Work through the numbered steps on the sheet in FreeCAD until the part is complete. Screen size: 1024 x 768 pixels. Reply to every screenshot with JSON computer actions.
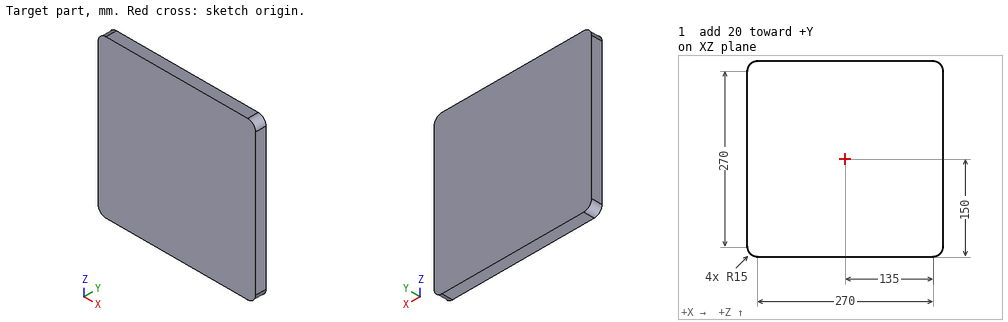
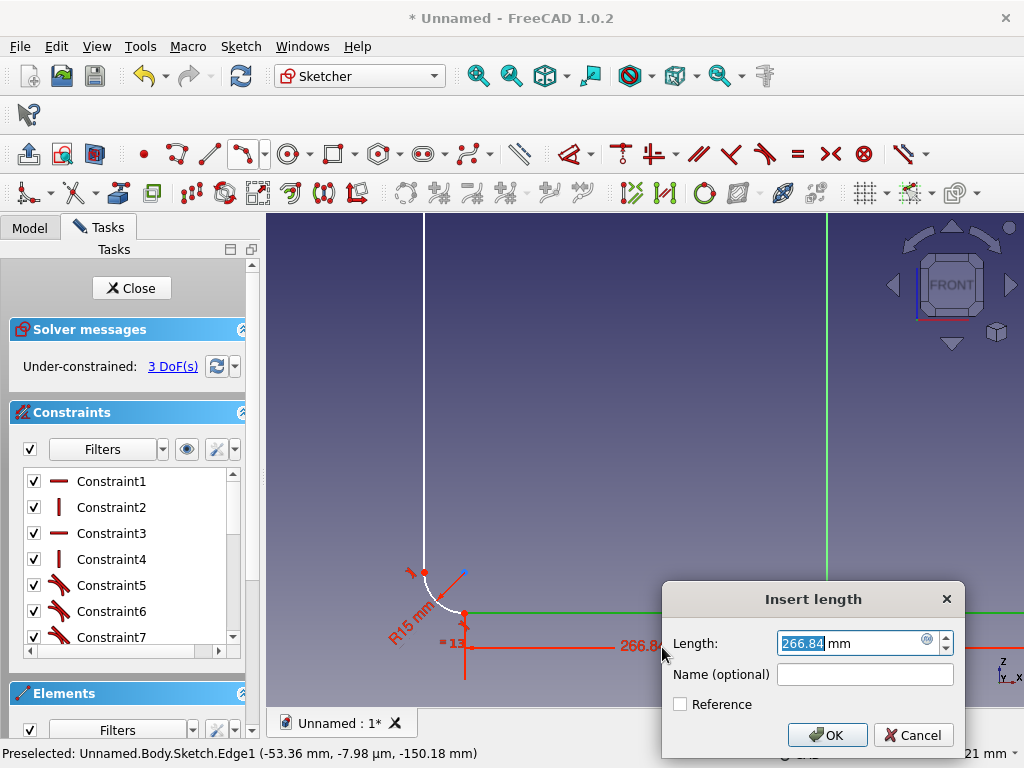
{"action": "type", "text": "270"}
{"action": "key", "text": "Return"}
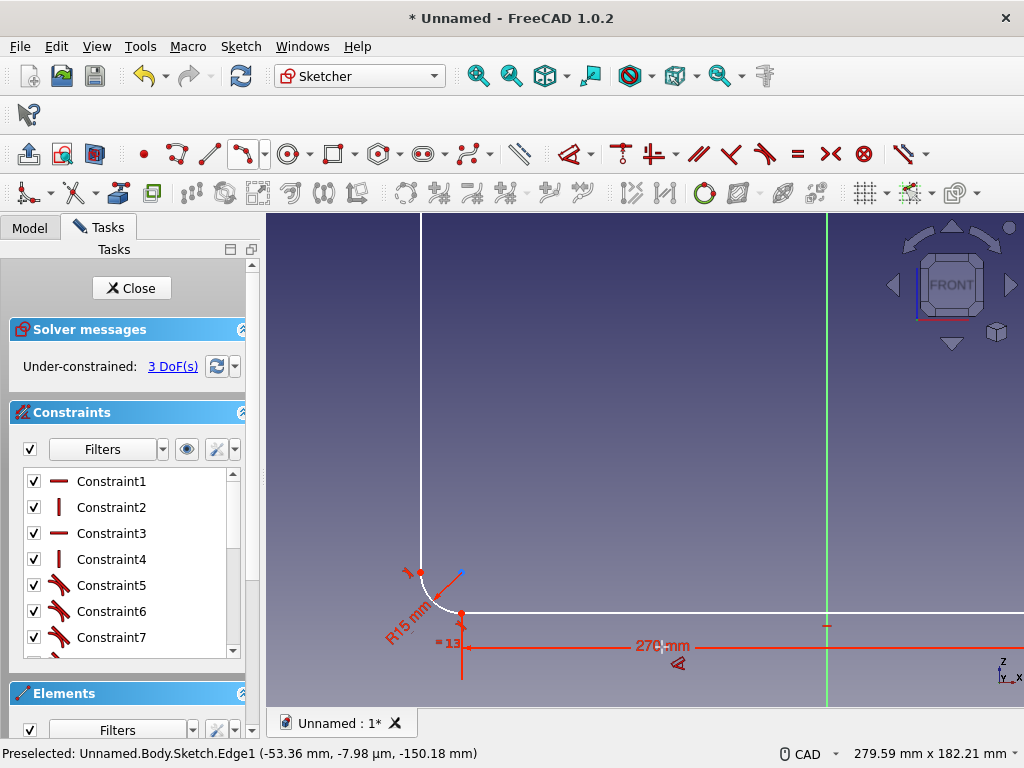
{"action": "left_click", "coordinate": [421, 353]}
{"action": "left_click", "coordinate": [387, 407]}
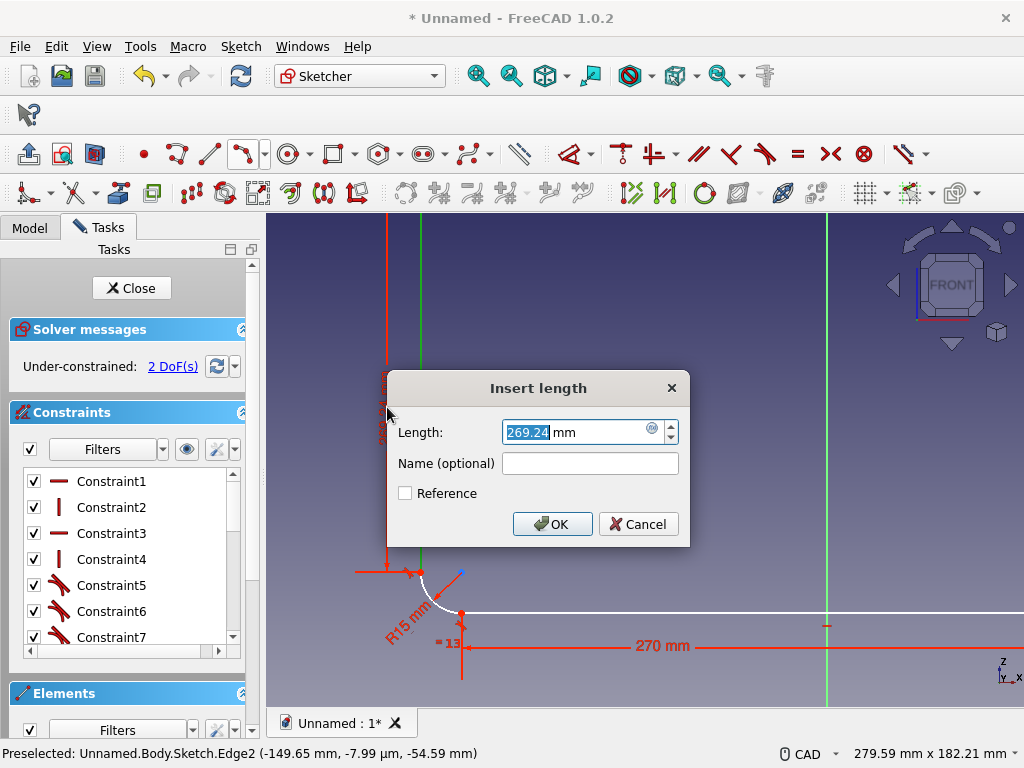
{"action": "type", "text": "270"}
{"action": "key", "text": "Return"}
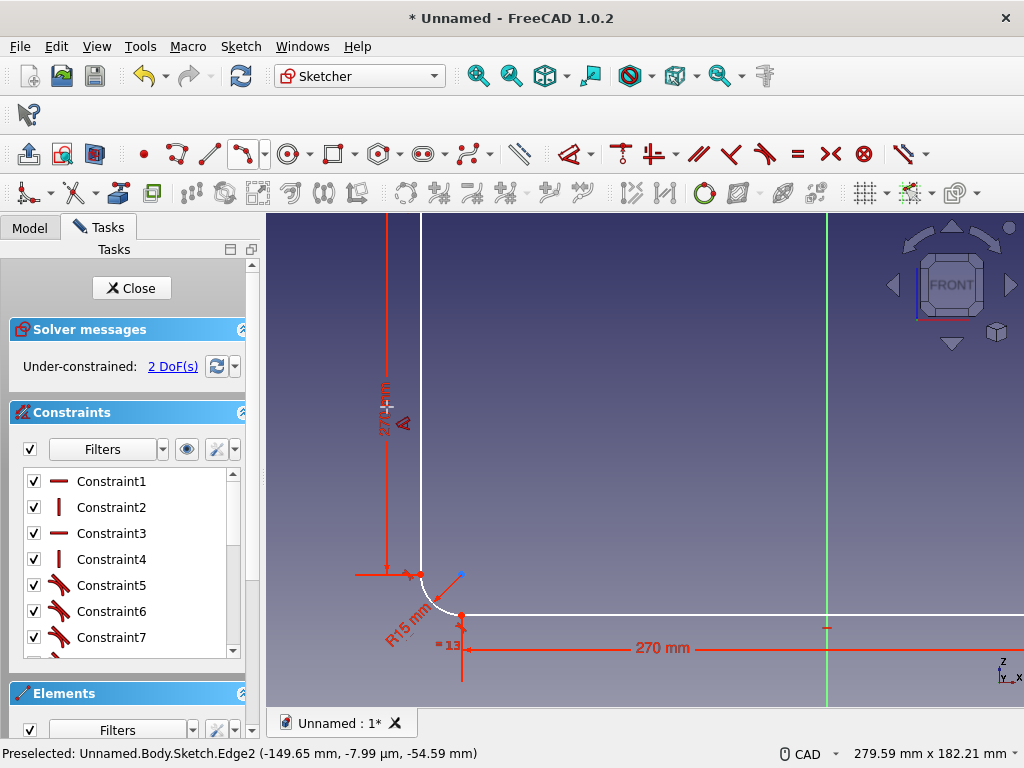
{"action": "scroll", "coordinate": [431, 608], "scroll_direction": "down", "scroll_amount": 5}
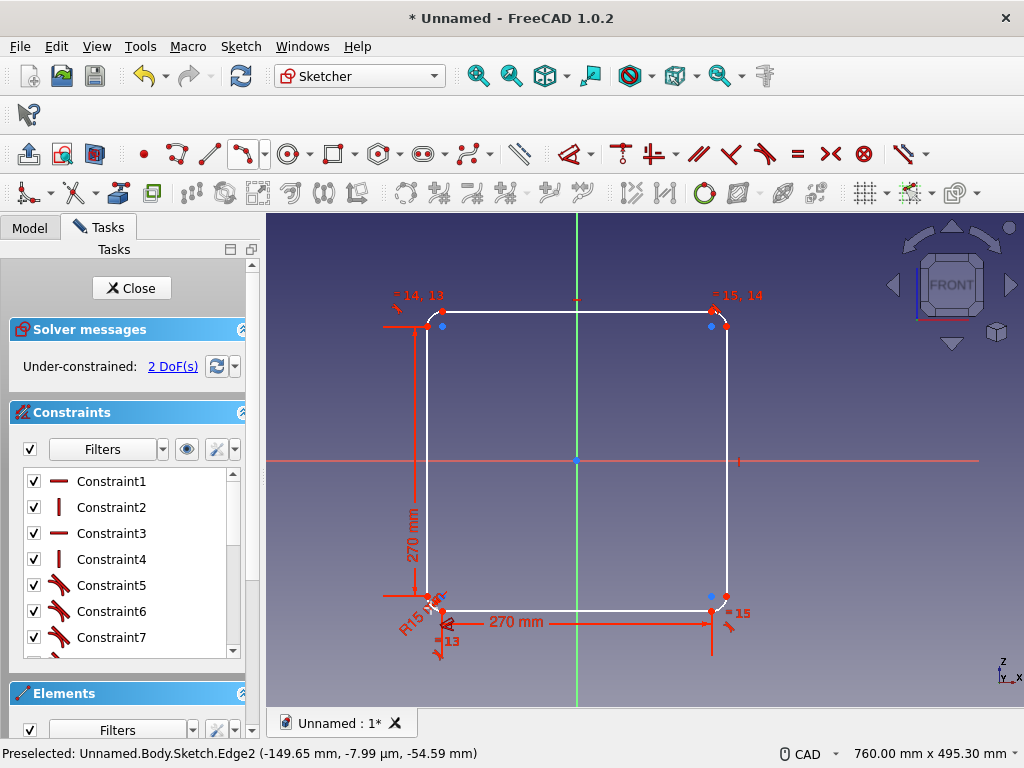
{"action": "left_click", "coordinate": [712, 611]}
{"action": "left_click", "coordinate": [644, 645]}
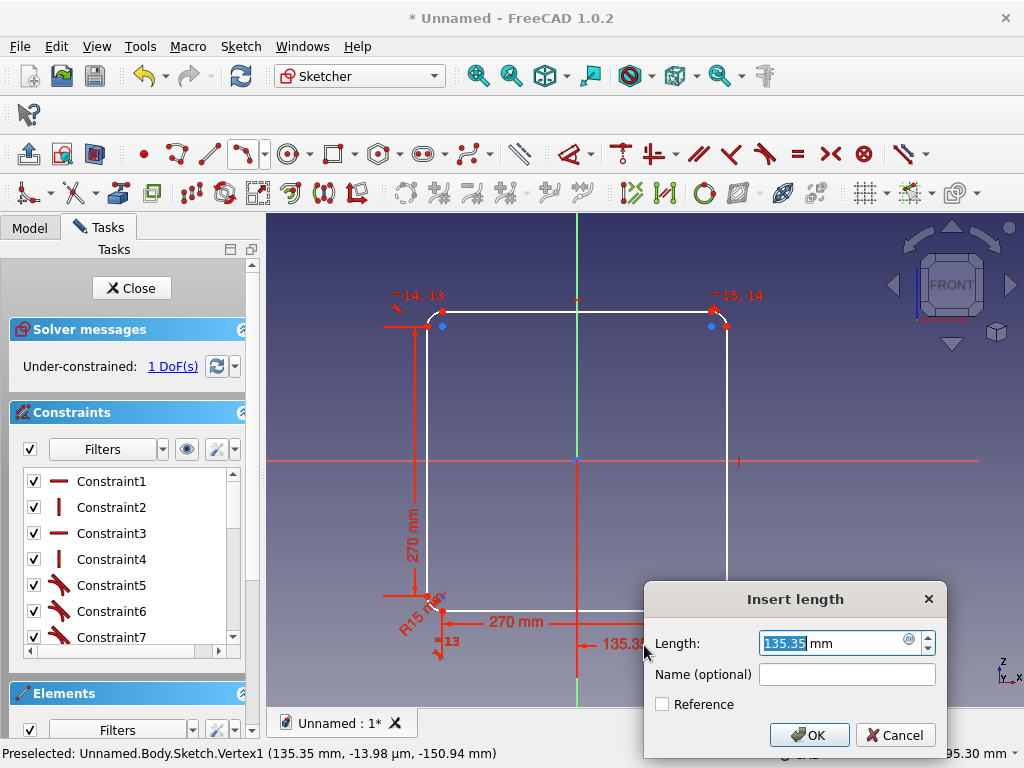
{"action": "type", "text": "135"}
{"action": "key", "text": "Return"}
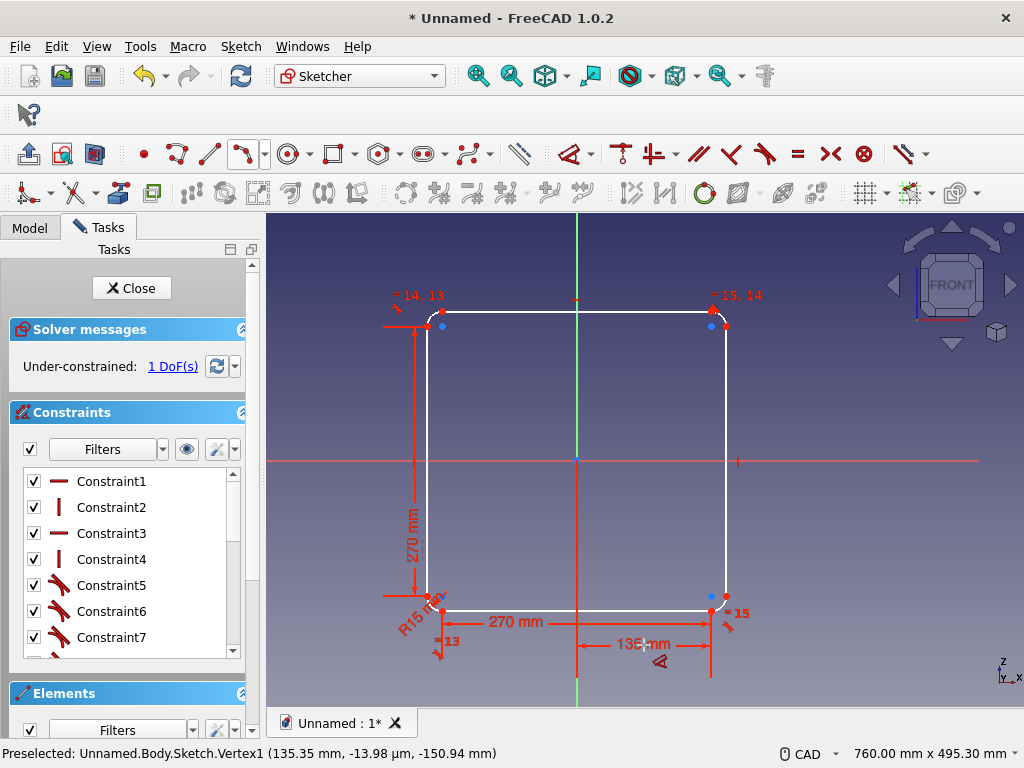
{"action": "left_click", "coordinate": [711, 611]}
{"action": "left_click", "coordinate": [745, 536]}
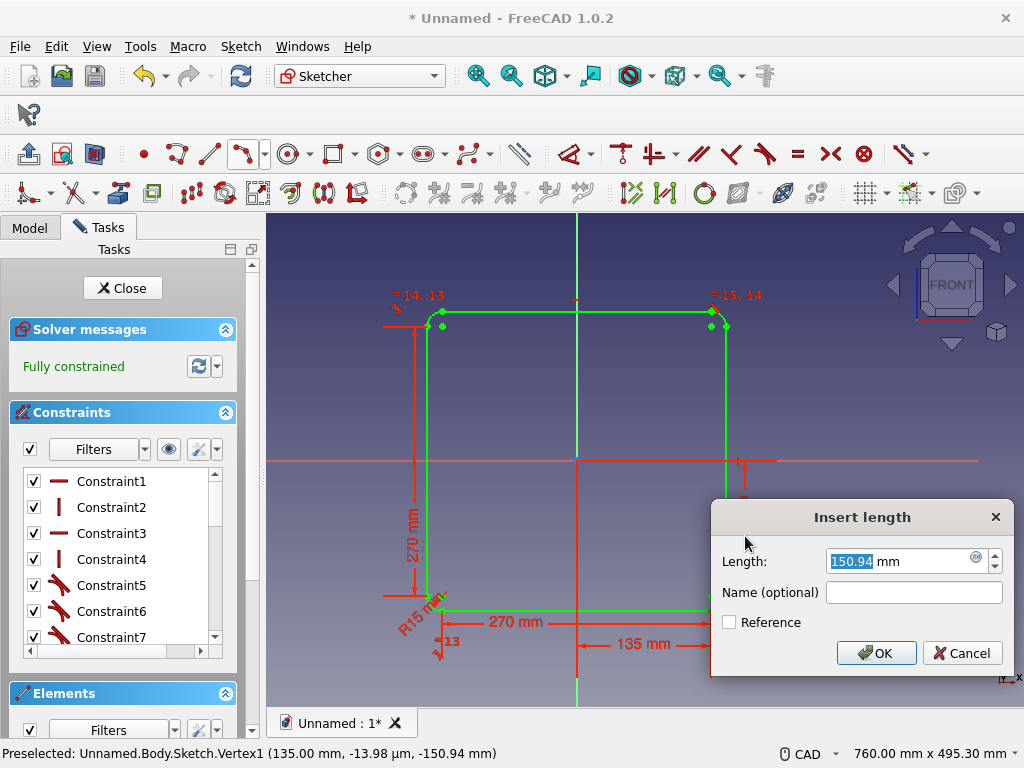
{"action": "type", "text": "150"}
{"action": "key", "text": "Return"}
{"action": "key", "text": "Escape"}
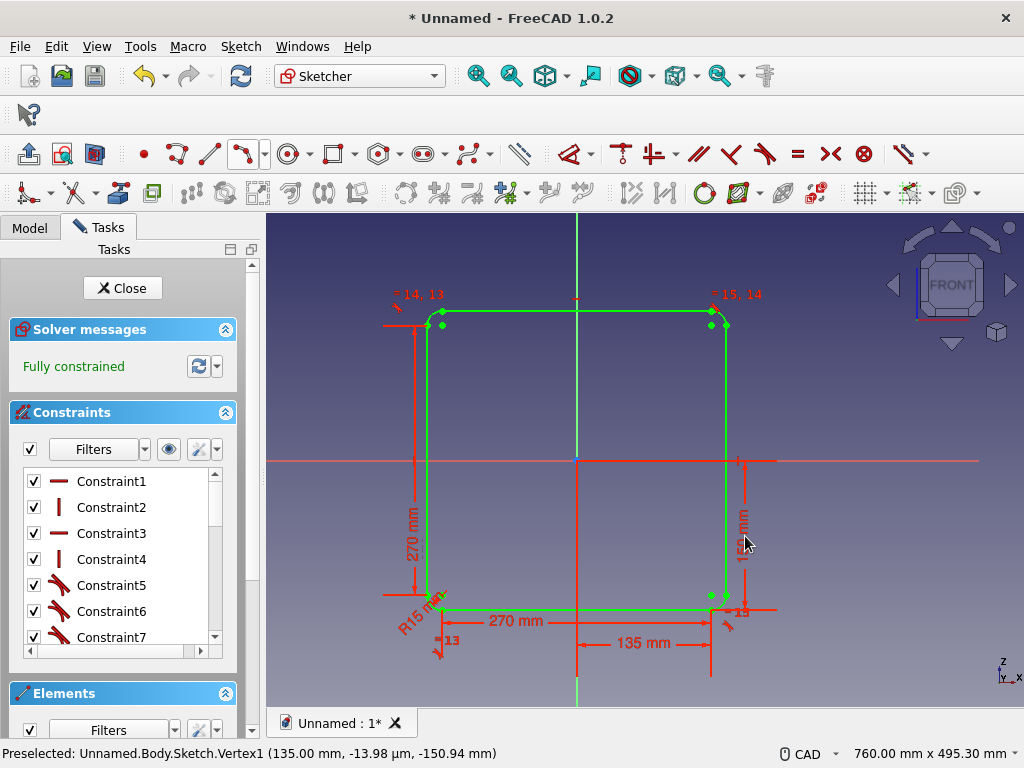
{"action": "left_click", "coordinate": [123, 288]}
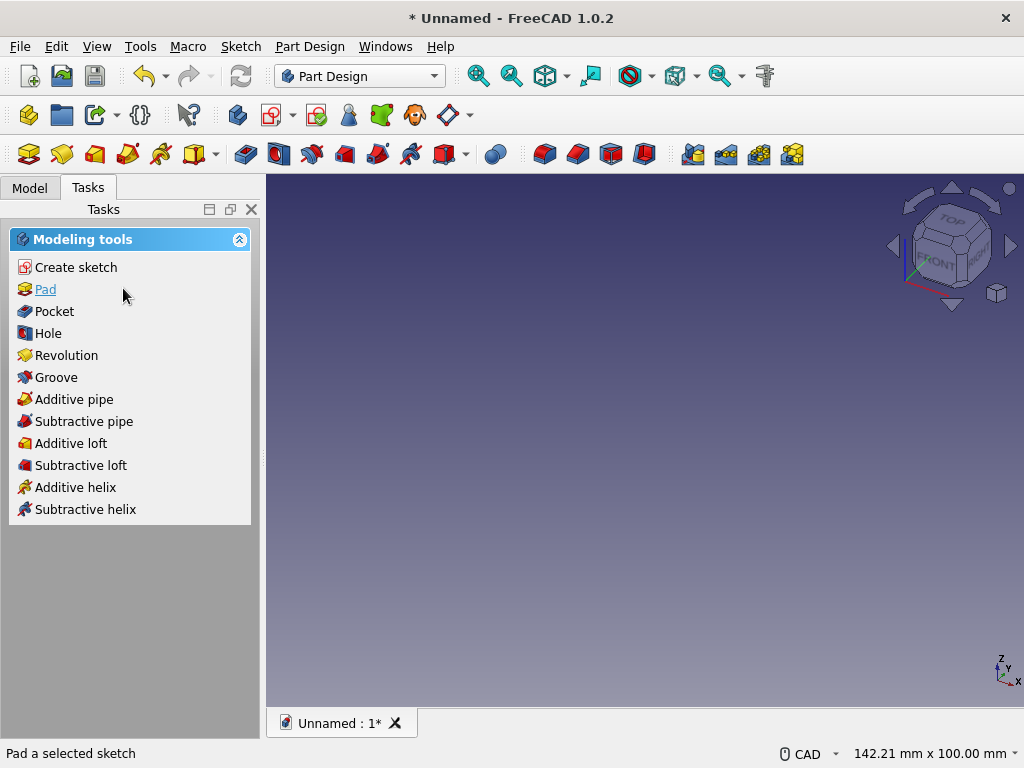
{"action": "left_click", "coordinate": [29, 154]}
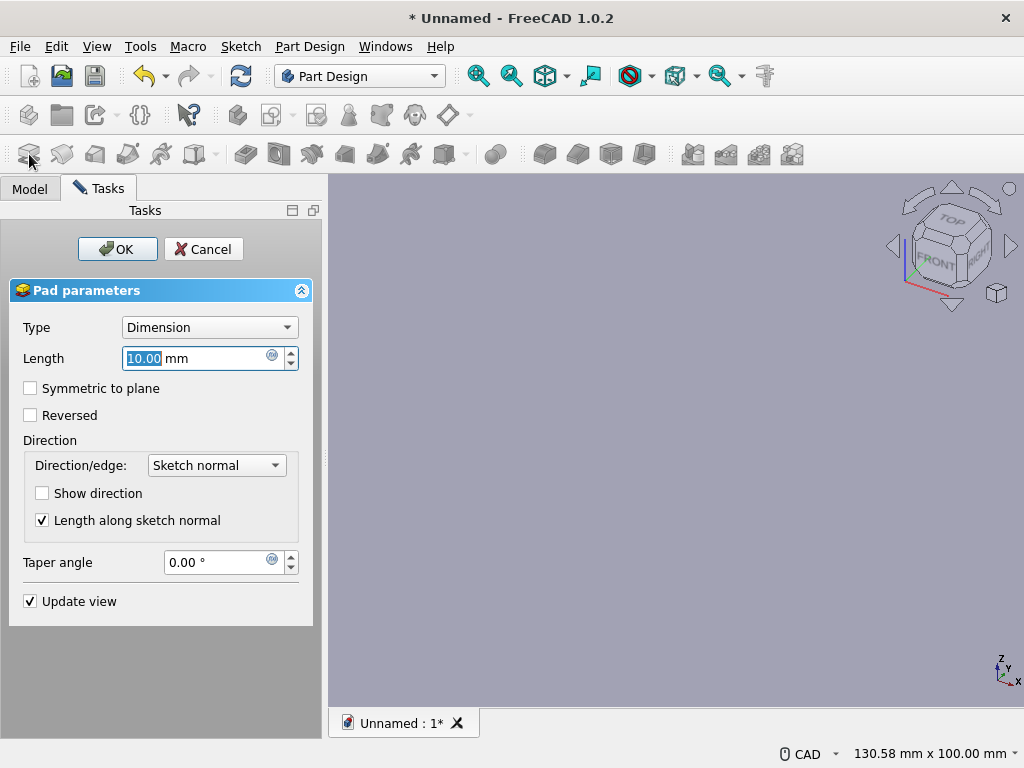
{"action": "type", "text": "20"}
{"action": "key", "text": "Tab"}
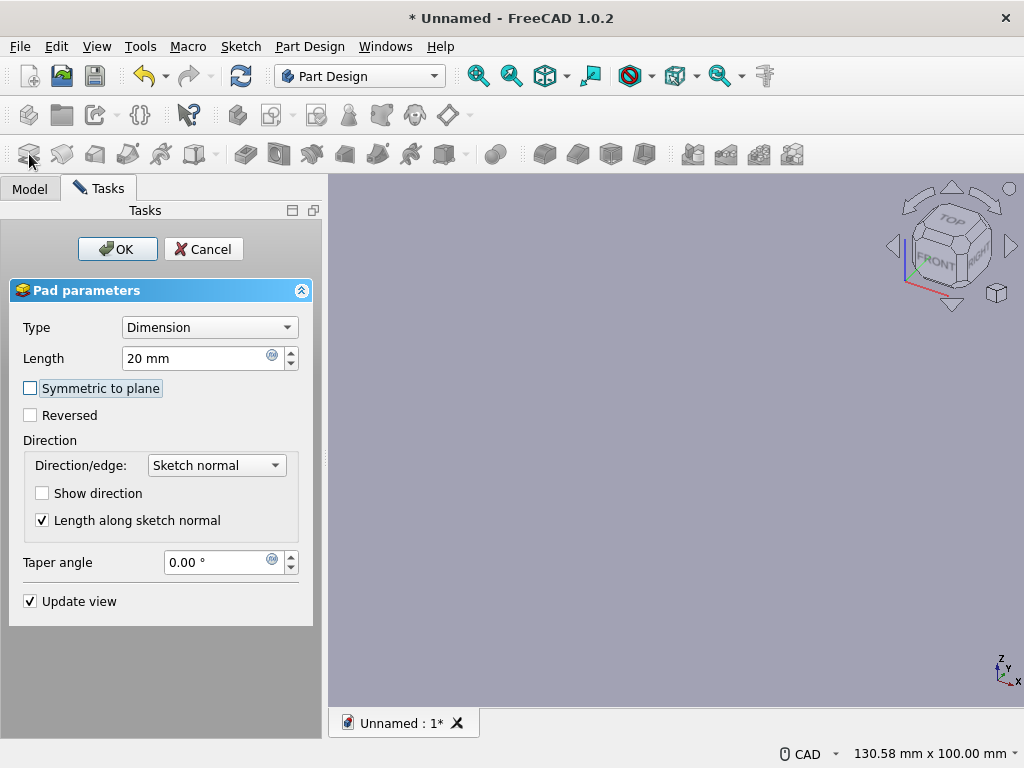
{"action": "left_click", "coordinate": [31, 415]}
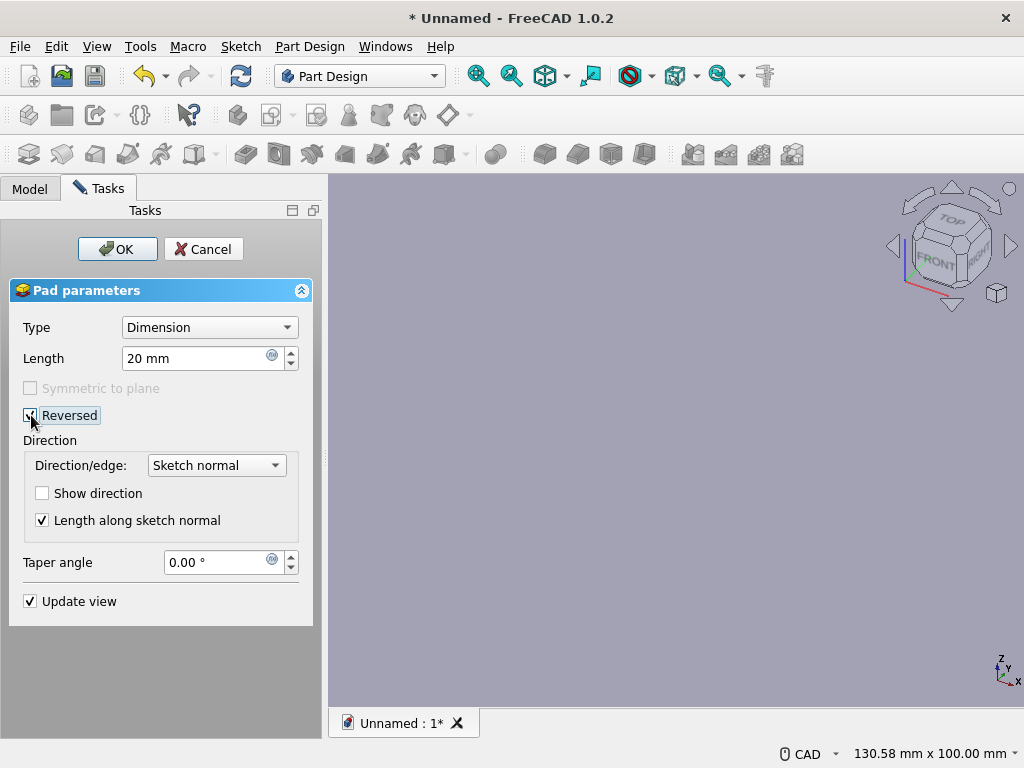
{"action": "left_click", "coordinate": [118, 249]}